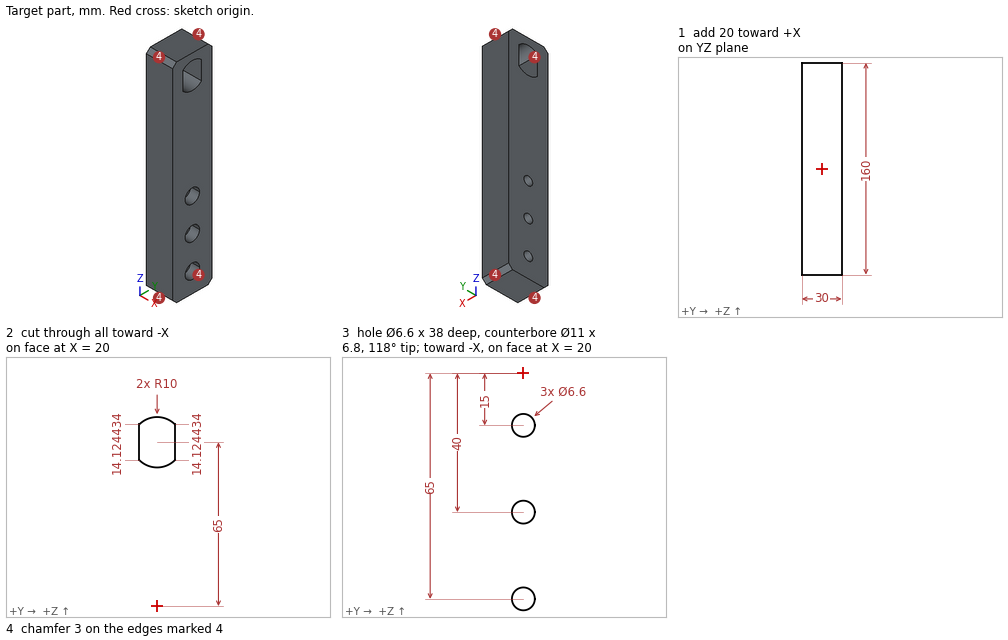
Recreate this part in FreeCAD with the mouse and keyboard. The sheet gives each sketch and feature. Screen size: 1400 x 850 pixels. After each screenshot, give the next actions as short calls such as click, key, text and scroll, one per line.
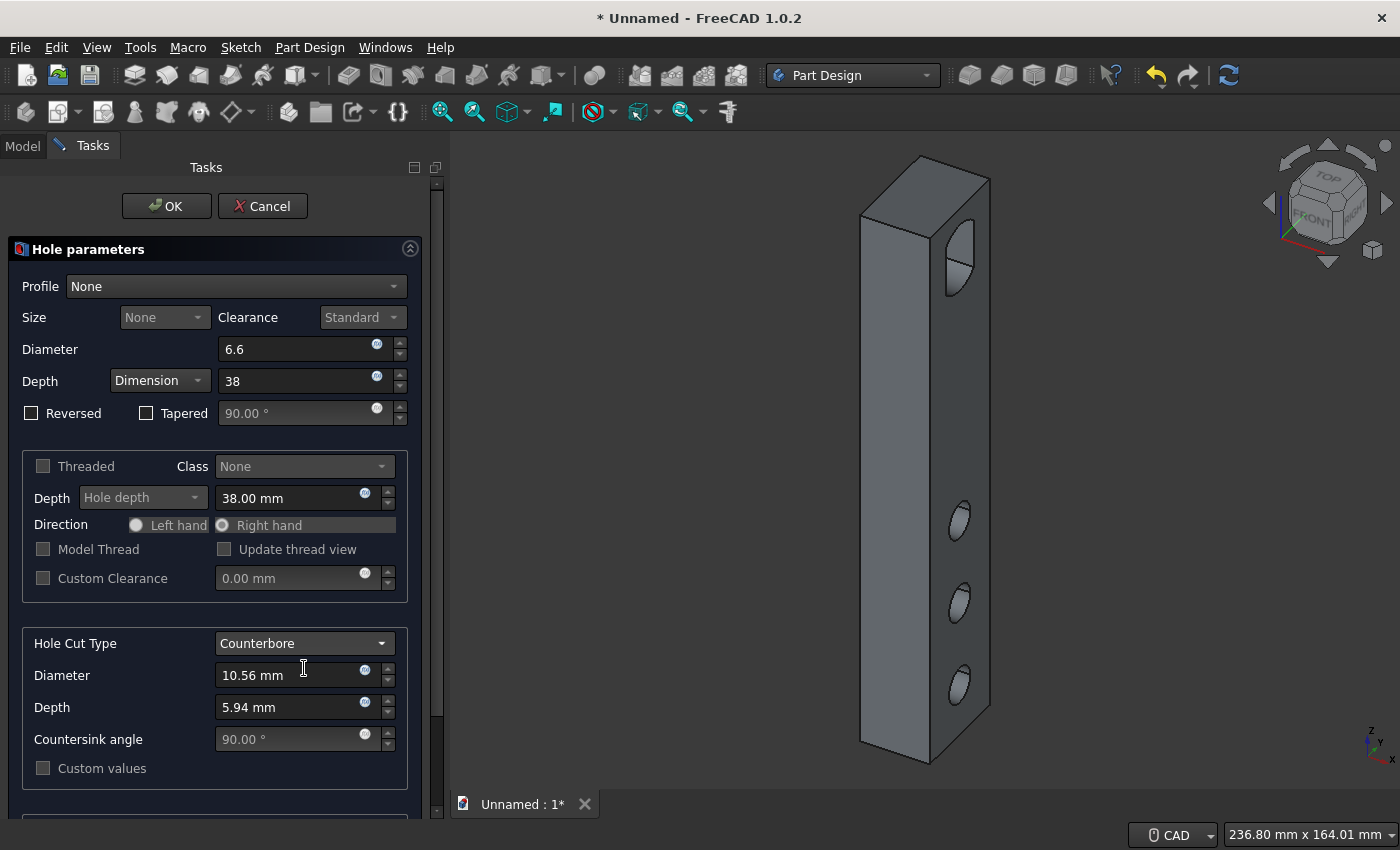
triple_click(298, 675)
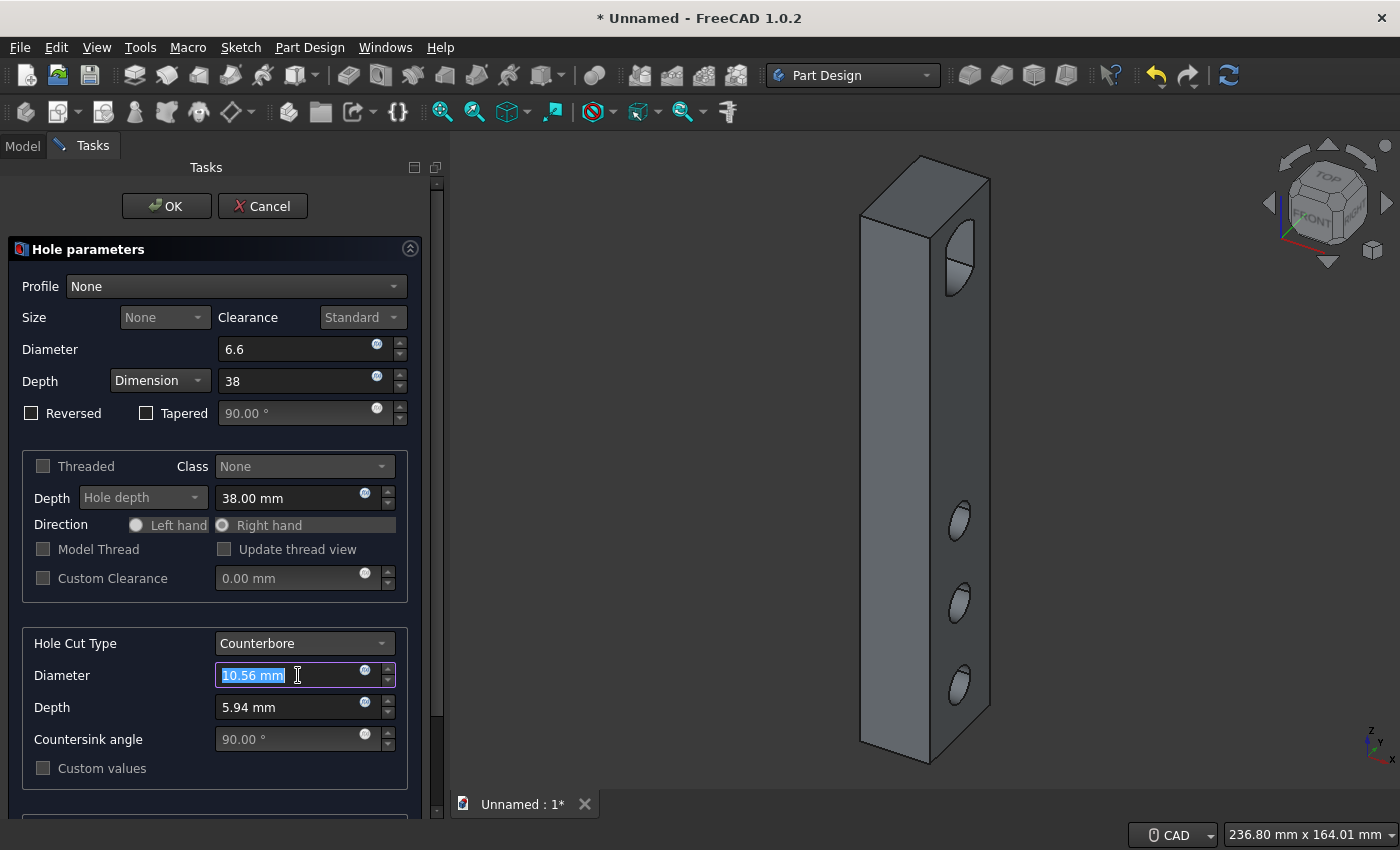
text(11)
key(Tab)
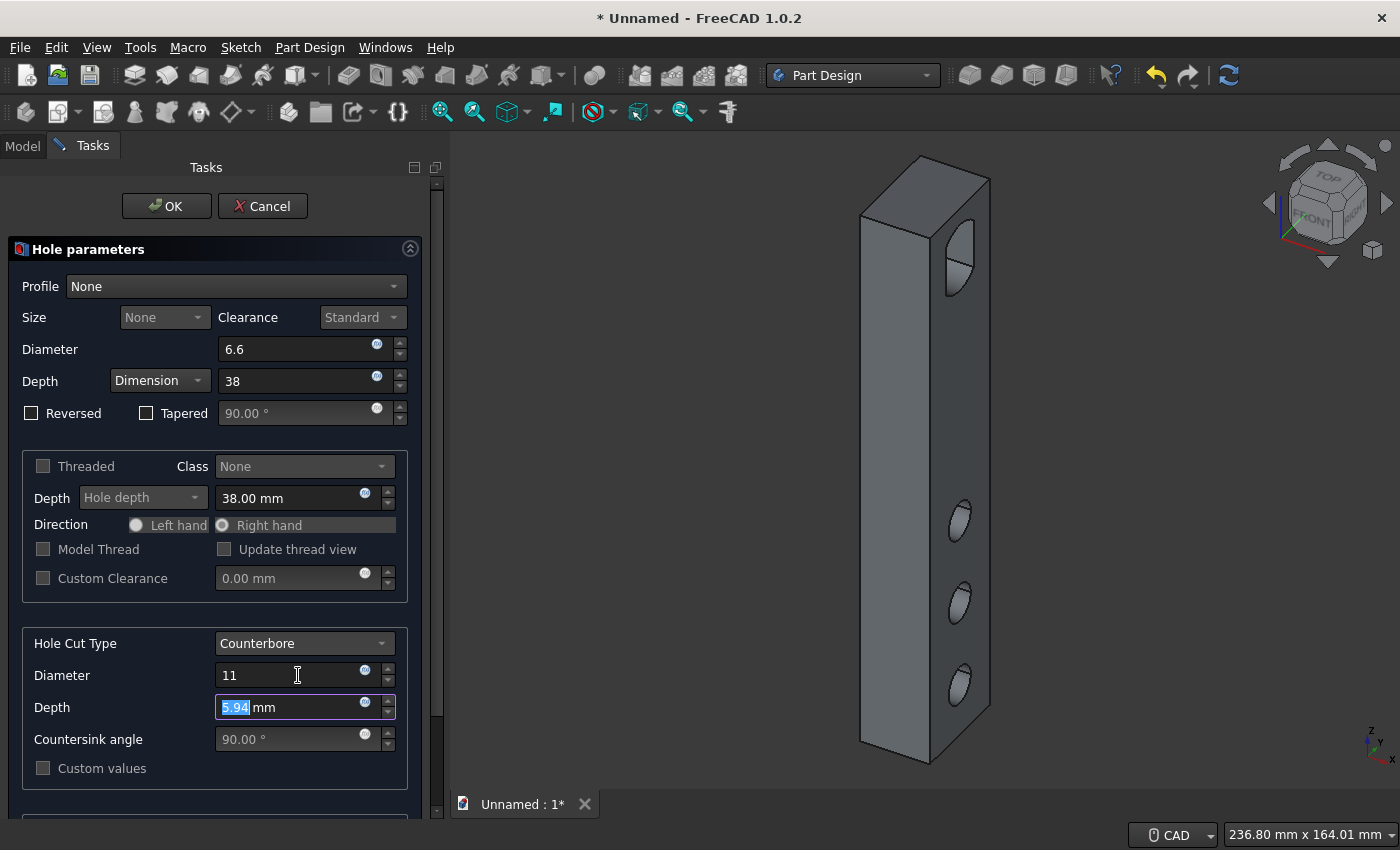
text(6.8)
key(Tab)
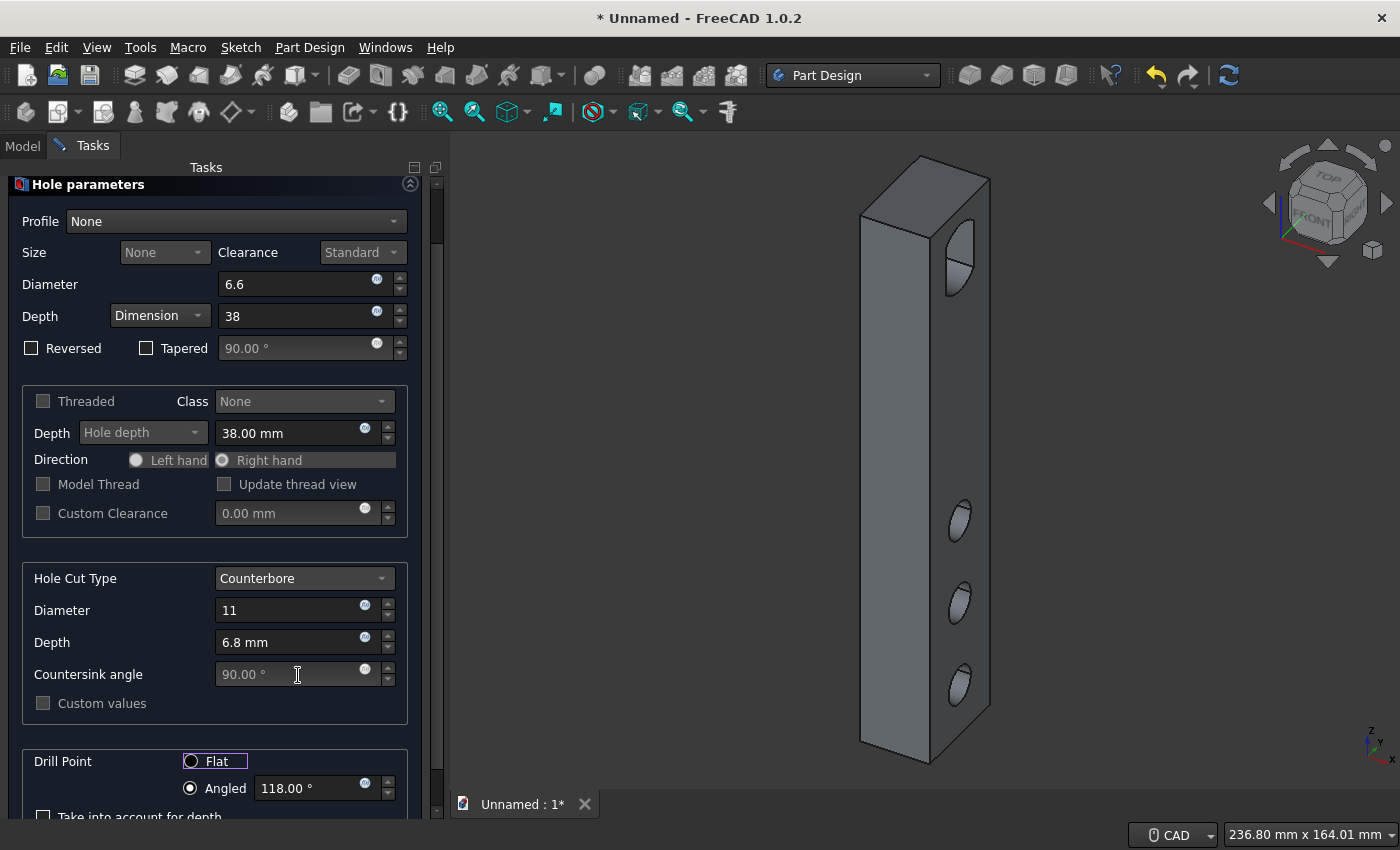
scroll(437, 498, up, 2)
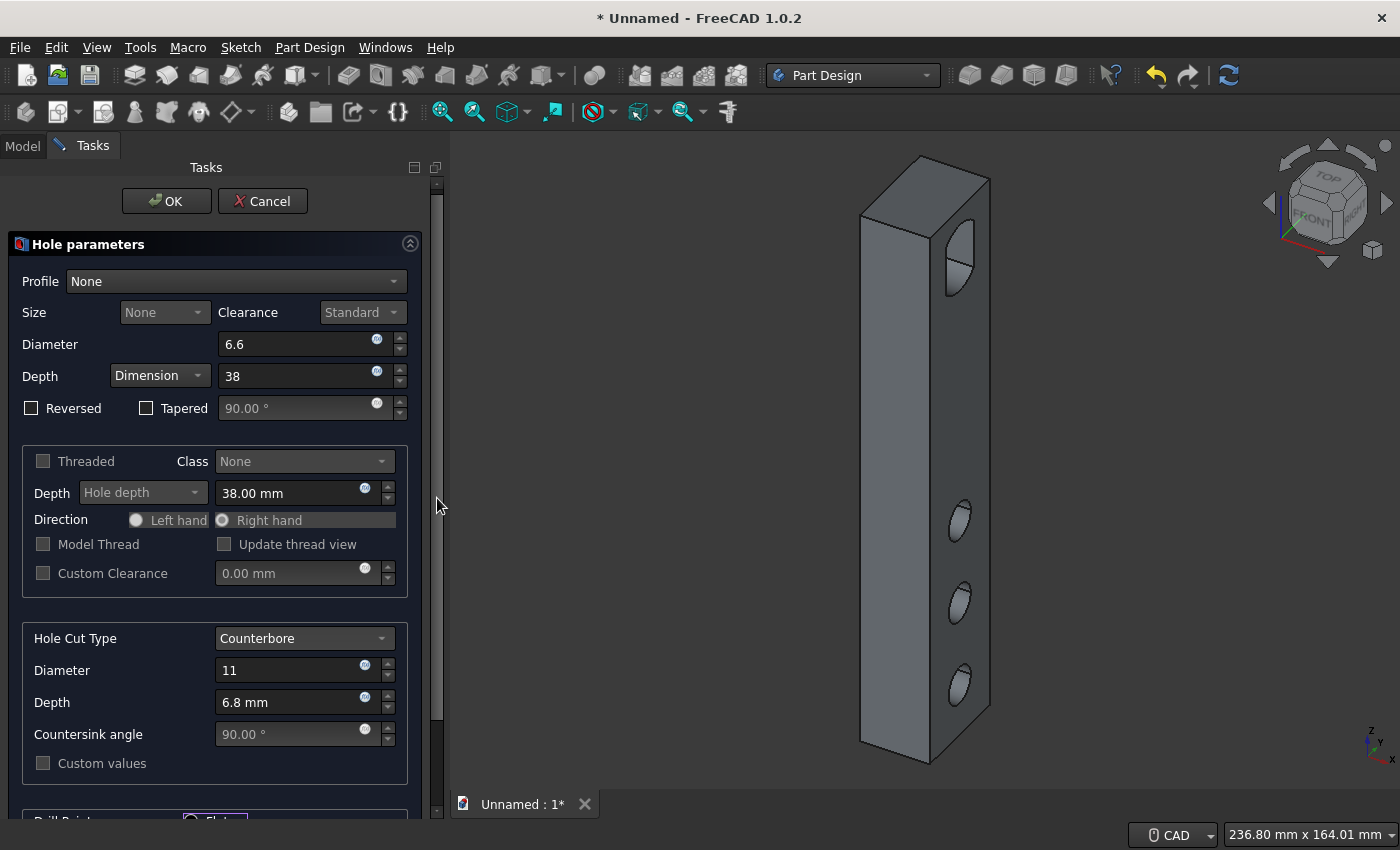
click(167, 206)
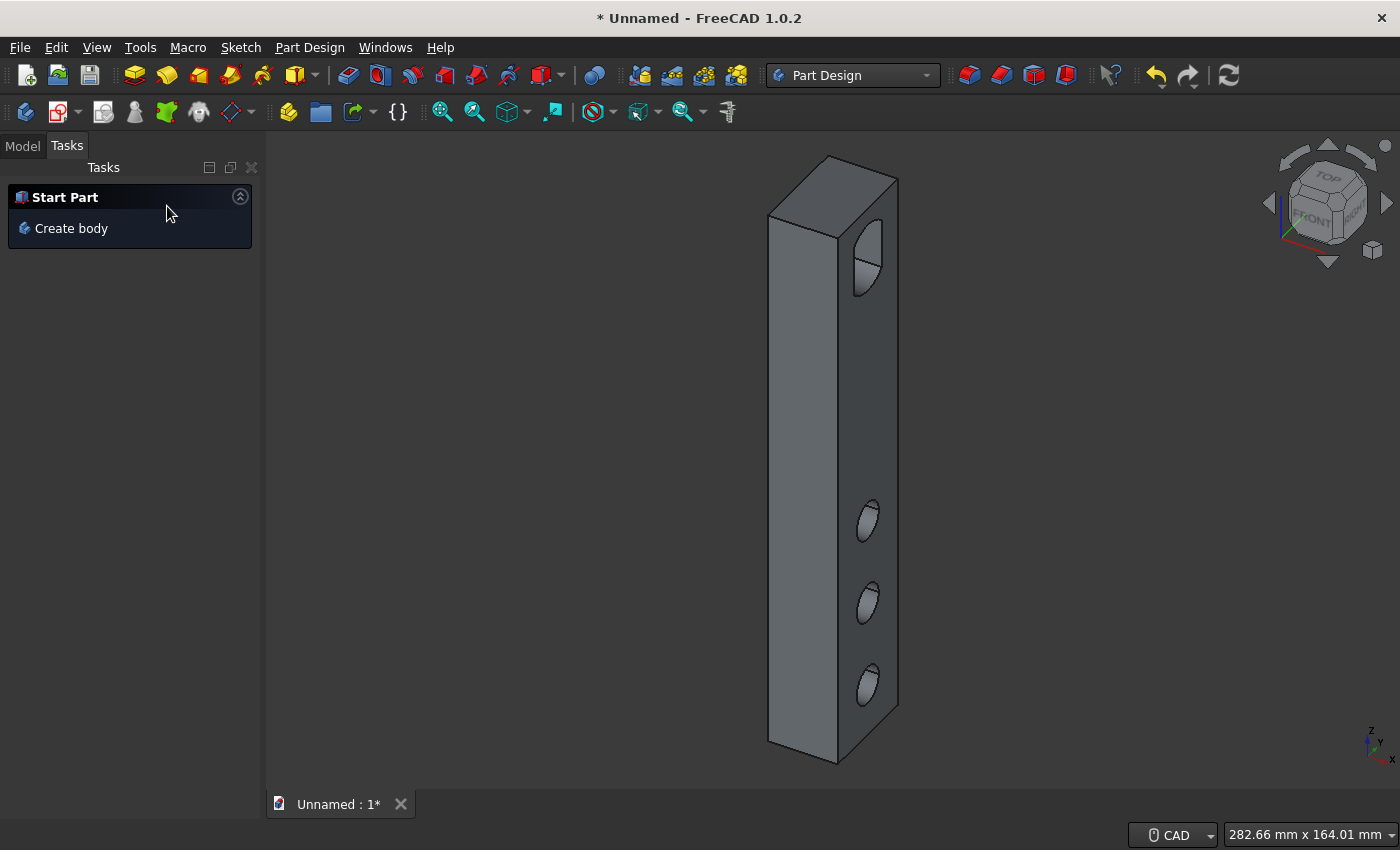
click(803, 226)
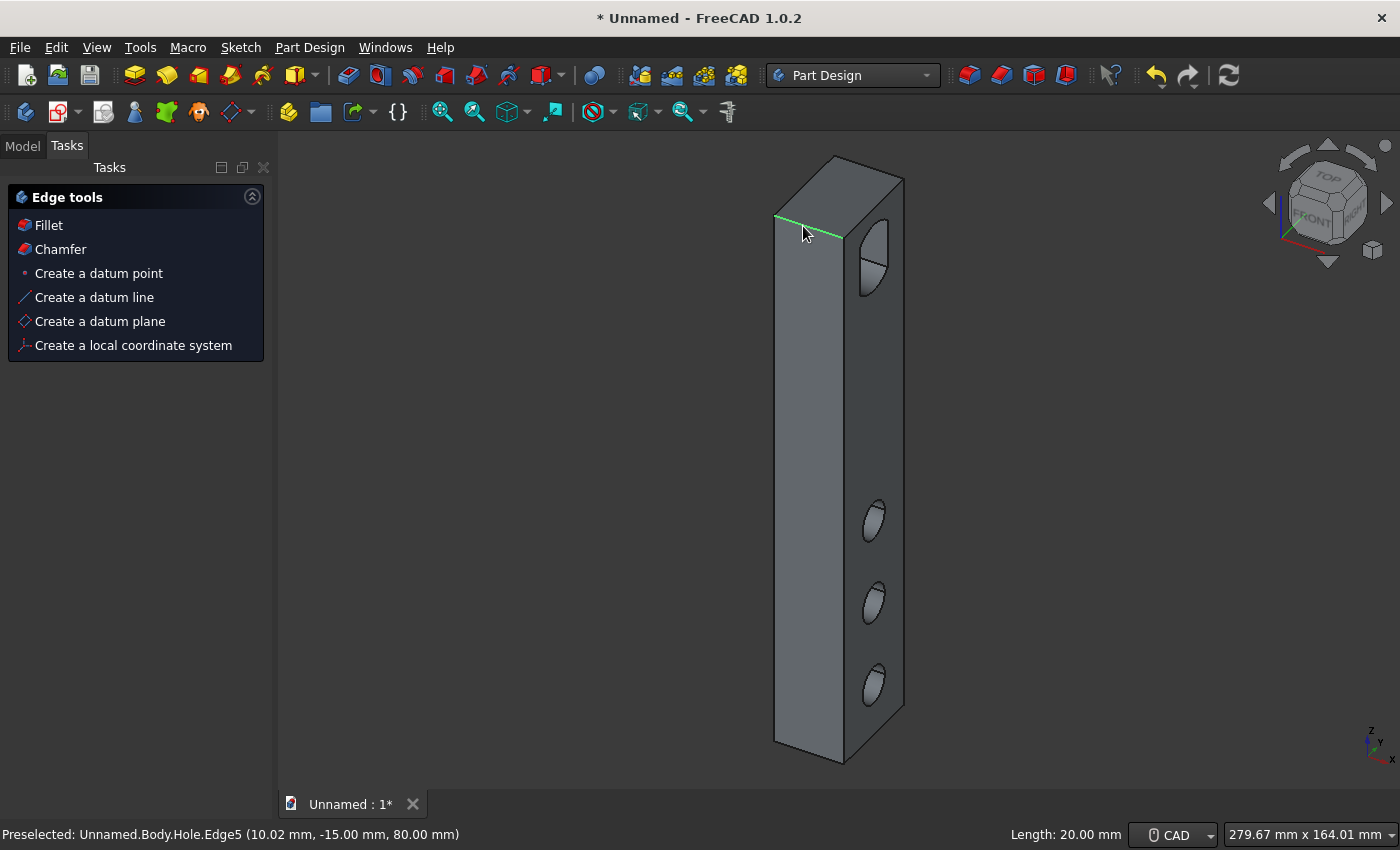
key(0)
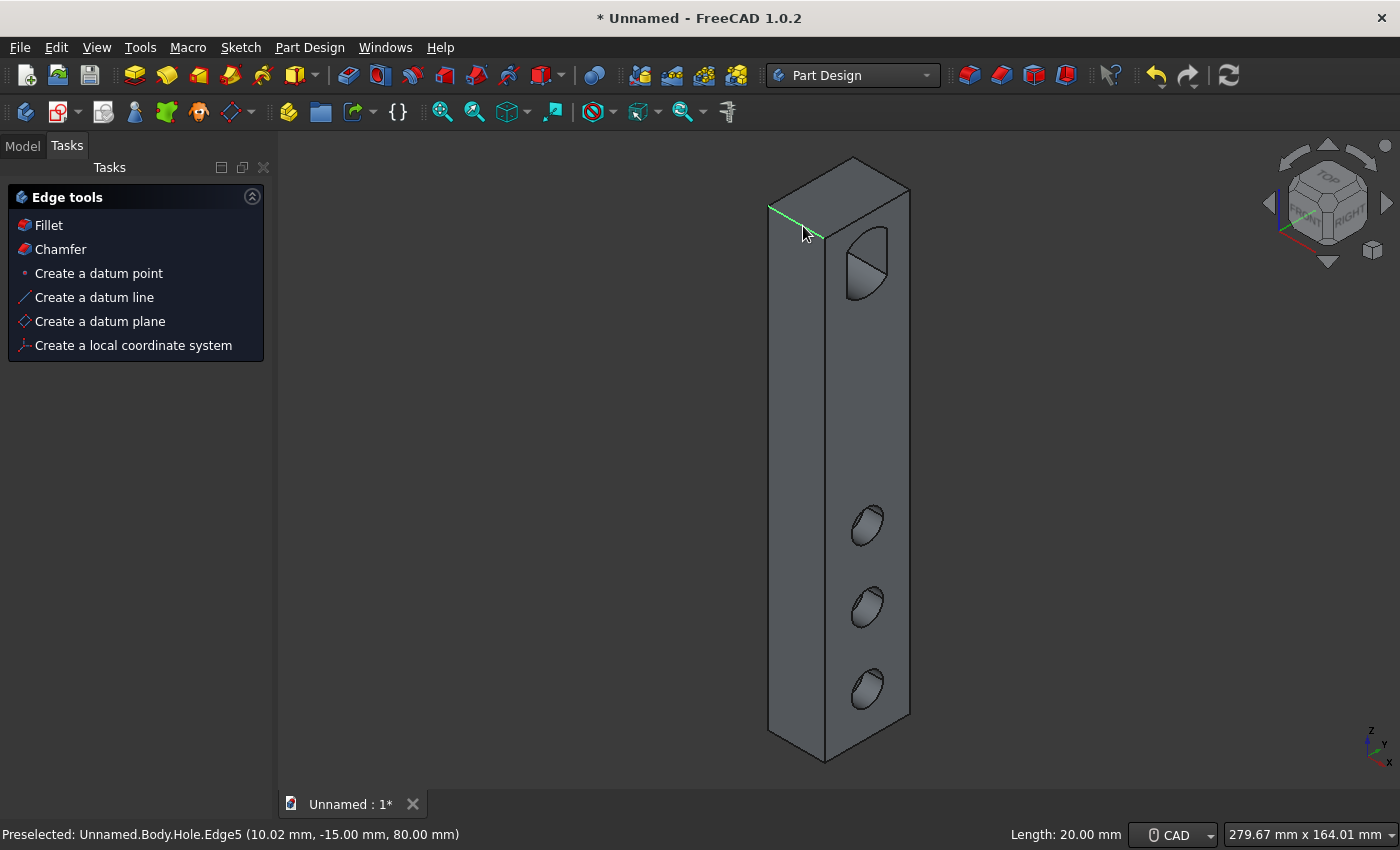
key(2)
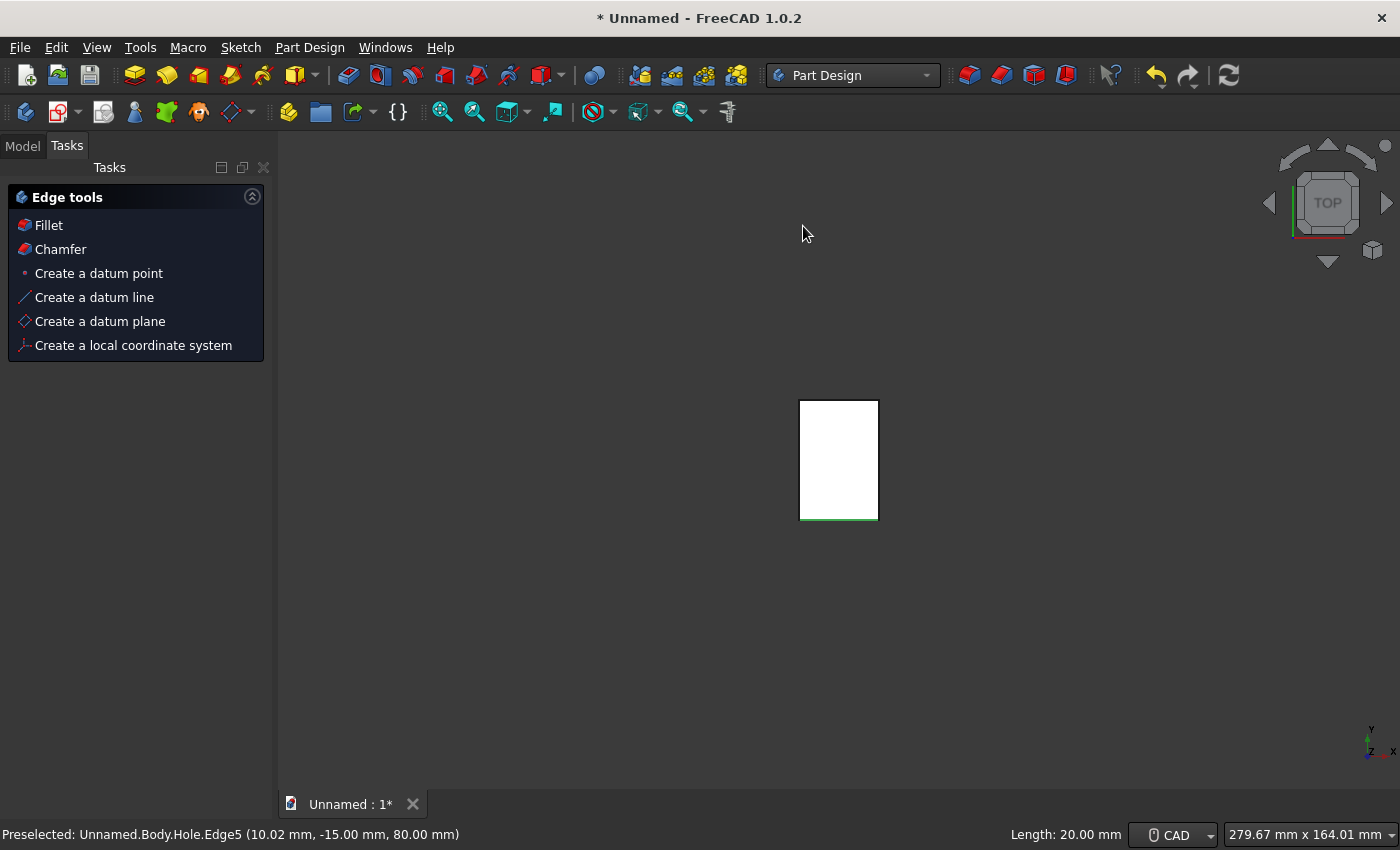
click(444, 112)